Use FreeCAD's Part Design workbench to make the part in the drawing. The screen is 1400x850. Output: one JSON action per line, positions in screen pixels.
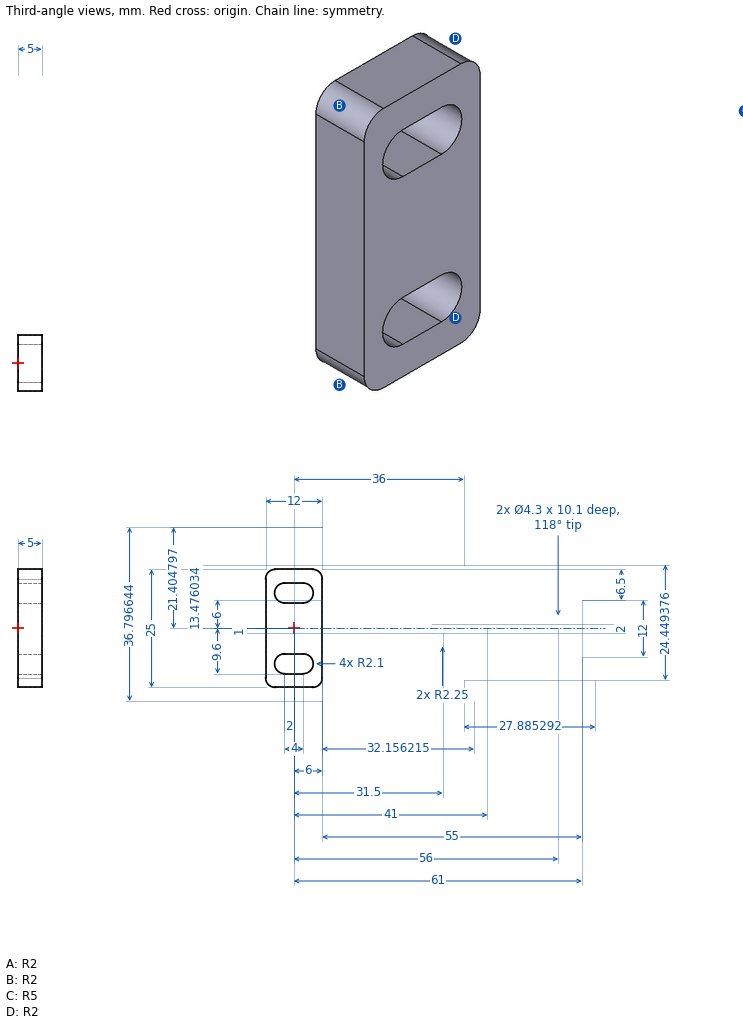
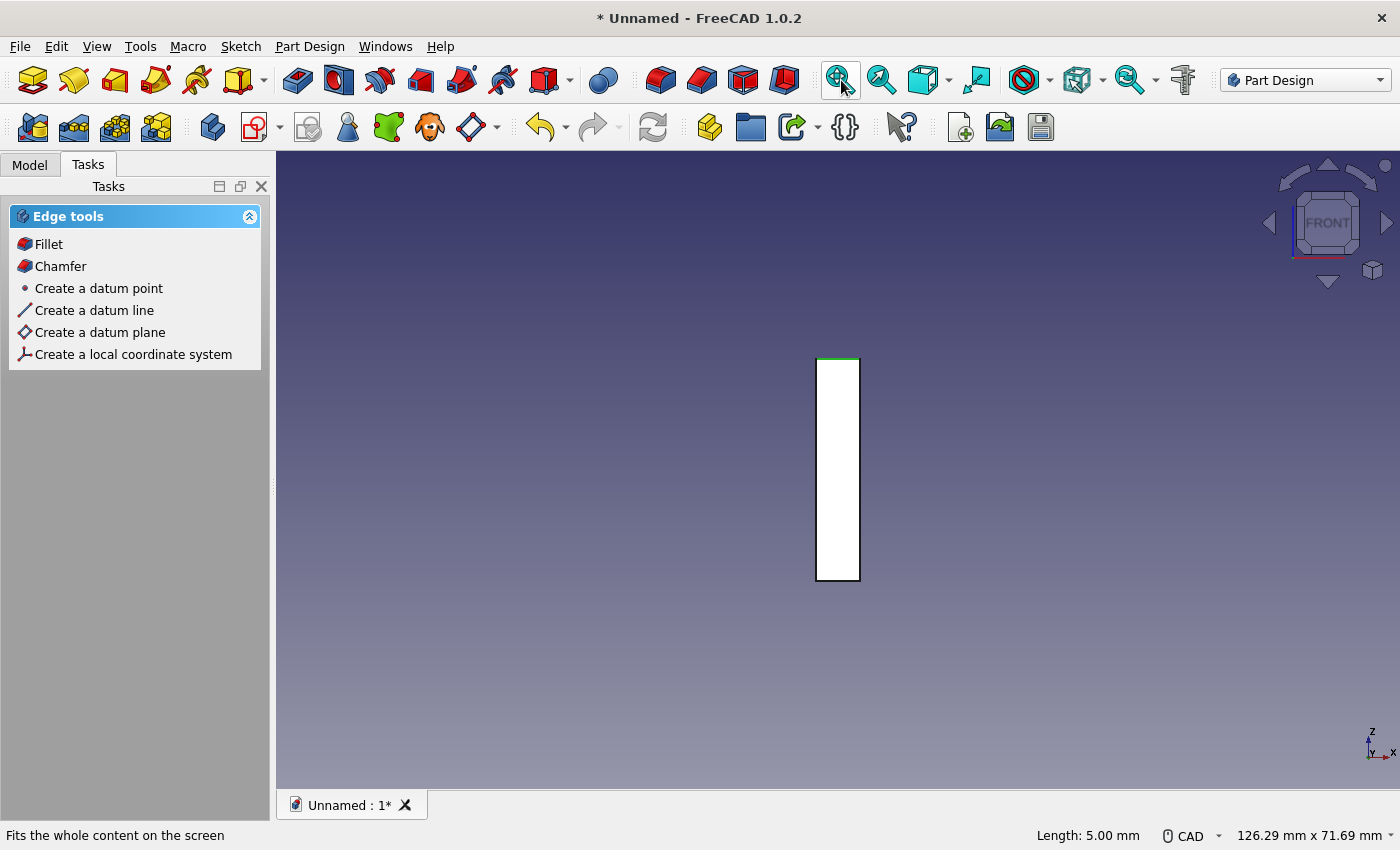
{"action": "left_click", "coordinate": [838, 580], "text": "ctrl"}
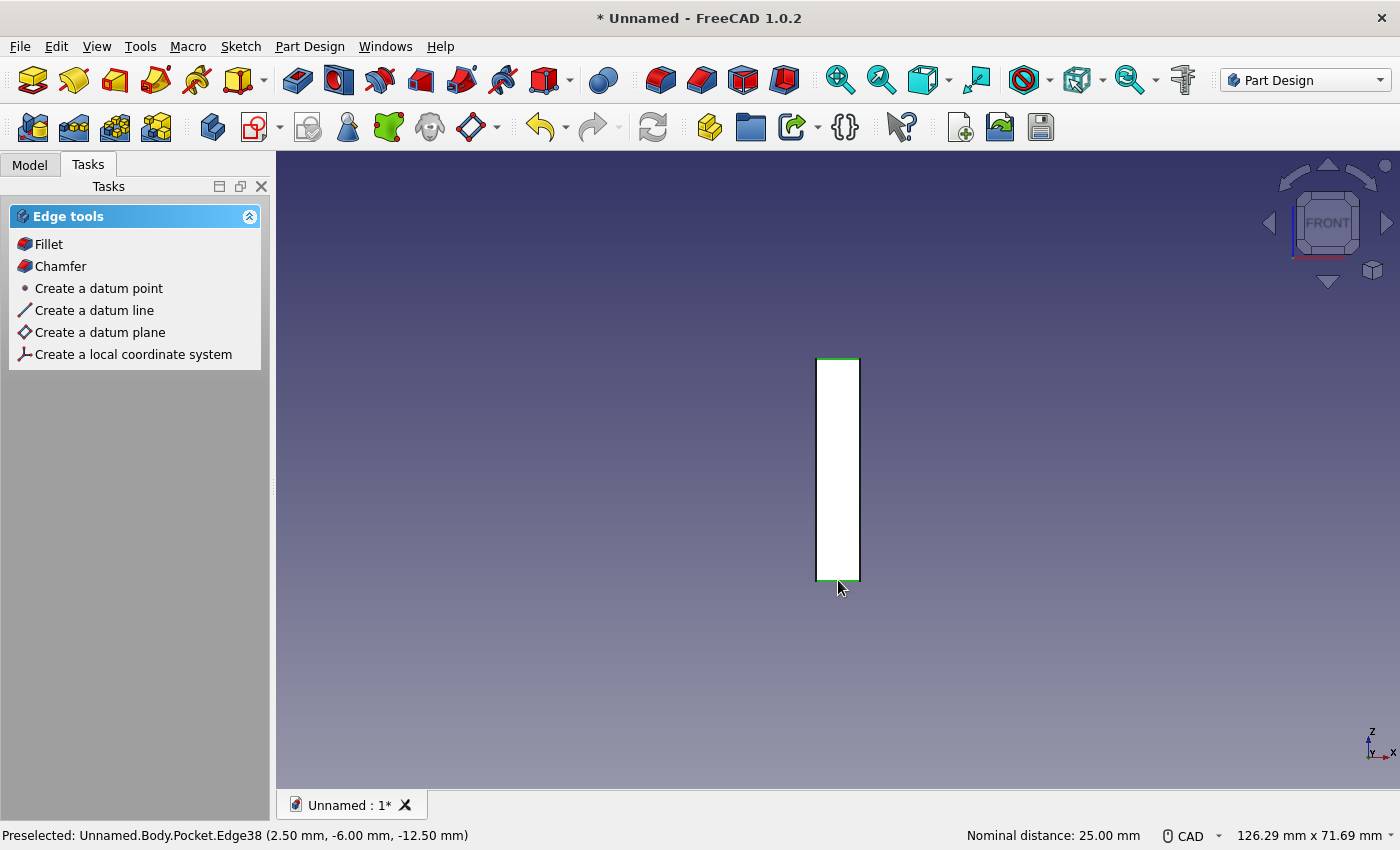
{"action": "left_click", "coordinate": [661, 80]}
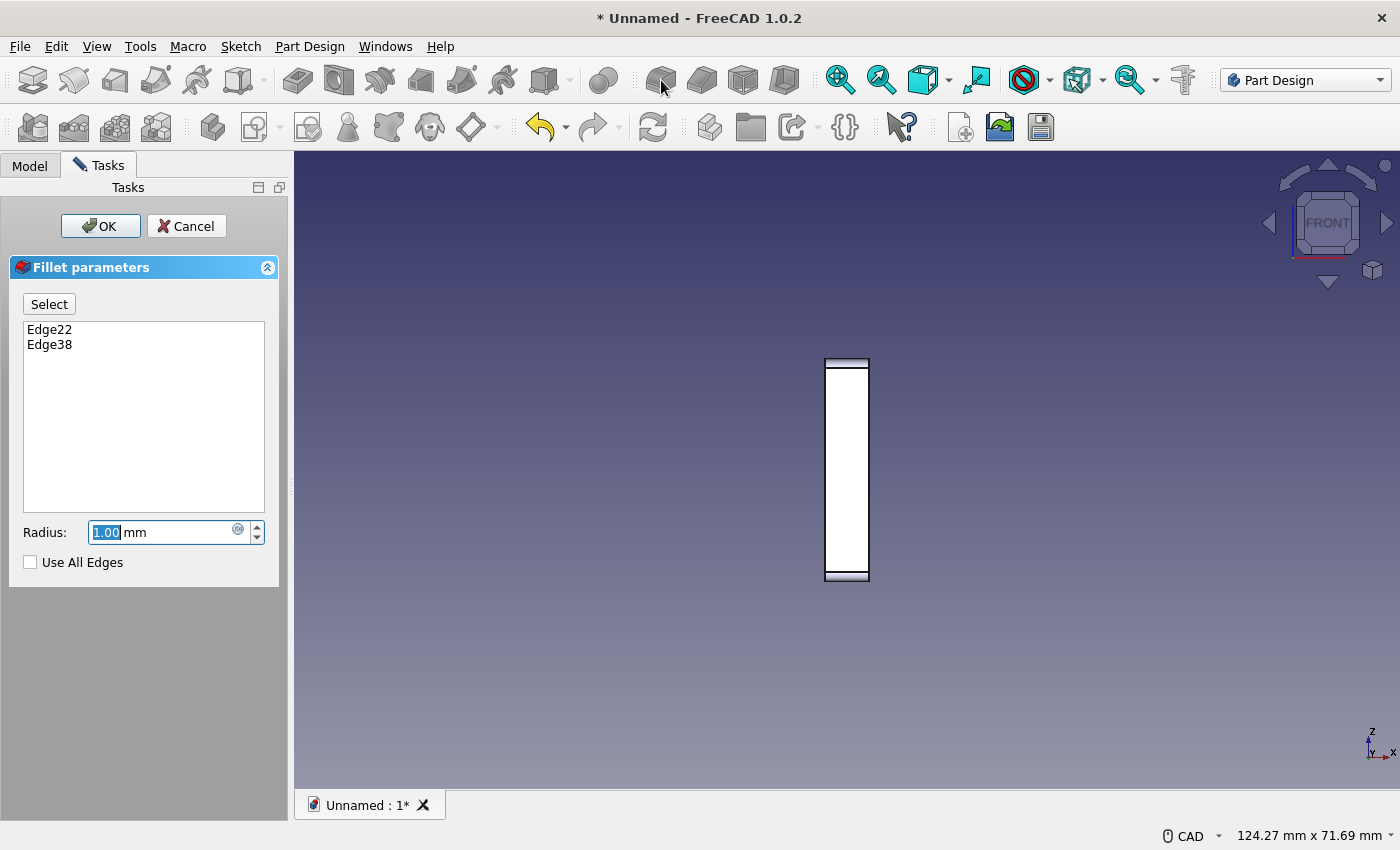
{"action": "type", "text": "2"}
{"action": "key", "text": "Tab"}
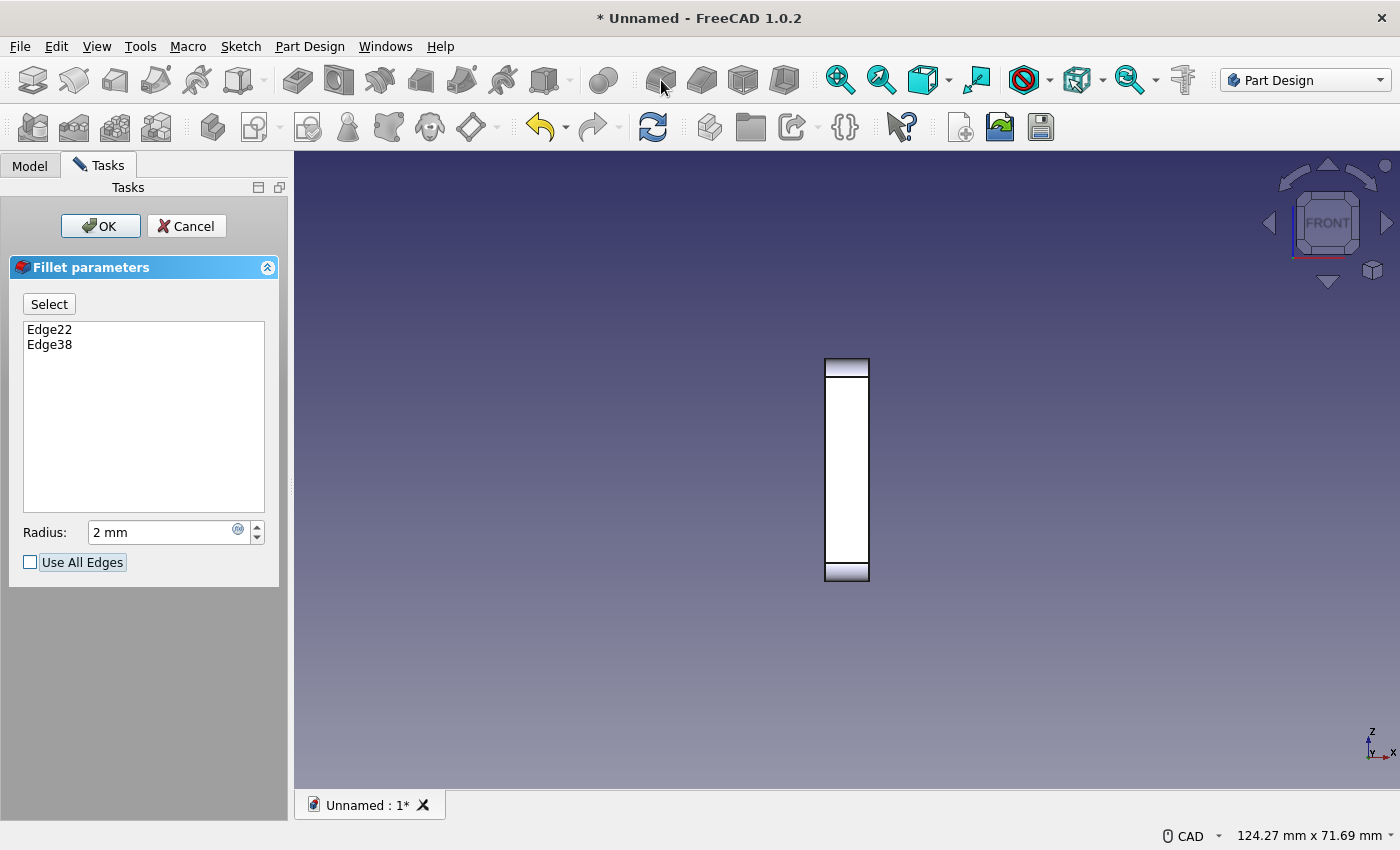
{"action": "left_click", "coordinate": [101, 226]}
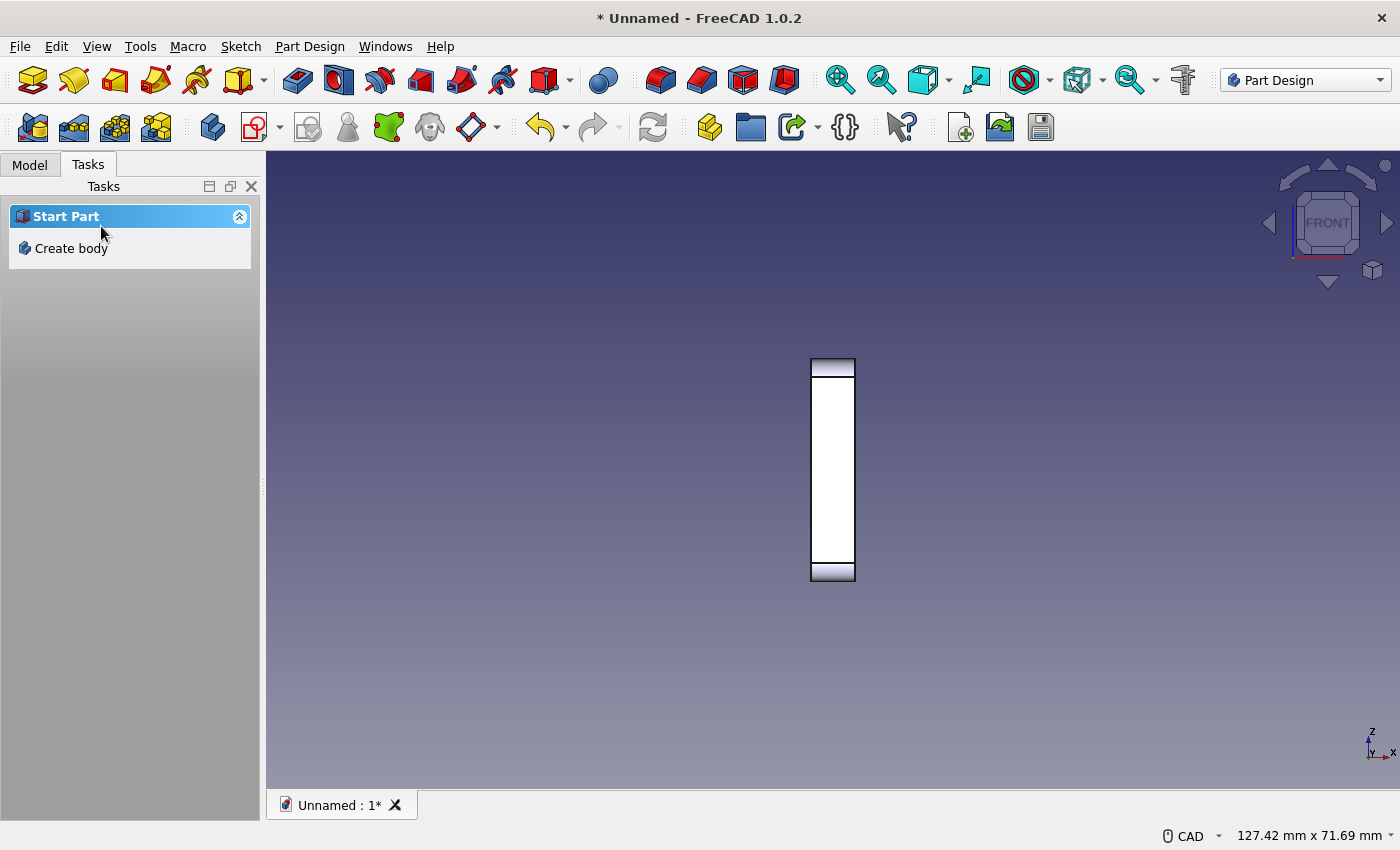
{"action": "left_click", "coordinate": [841, 80]}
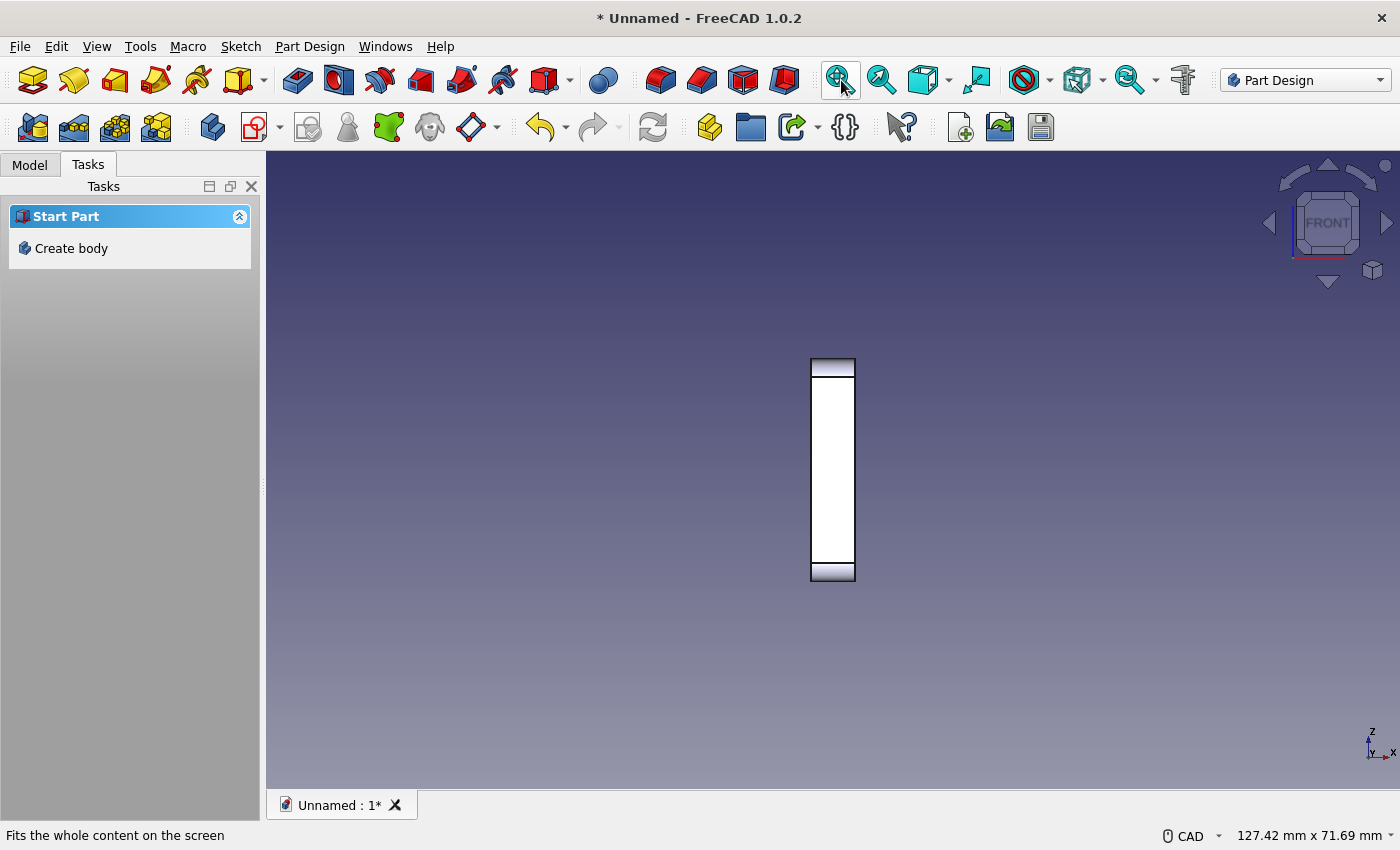
{"action": "left_click", "coordinate": [254, 128]}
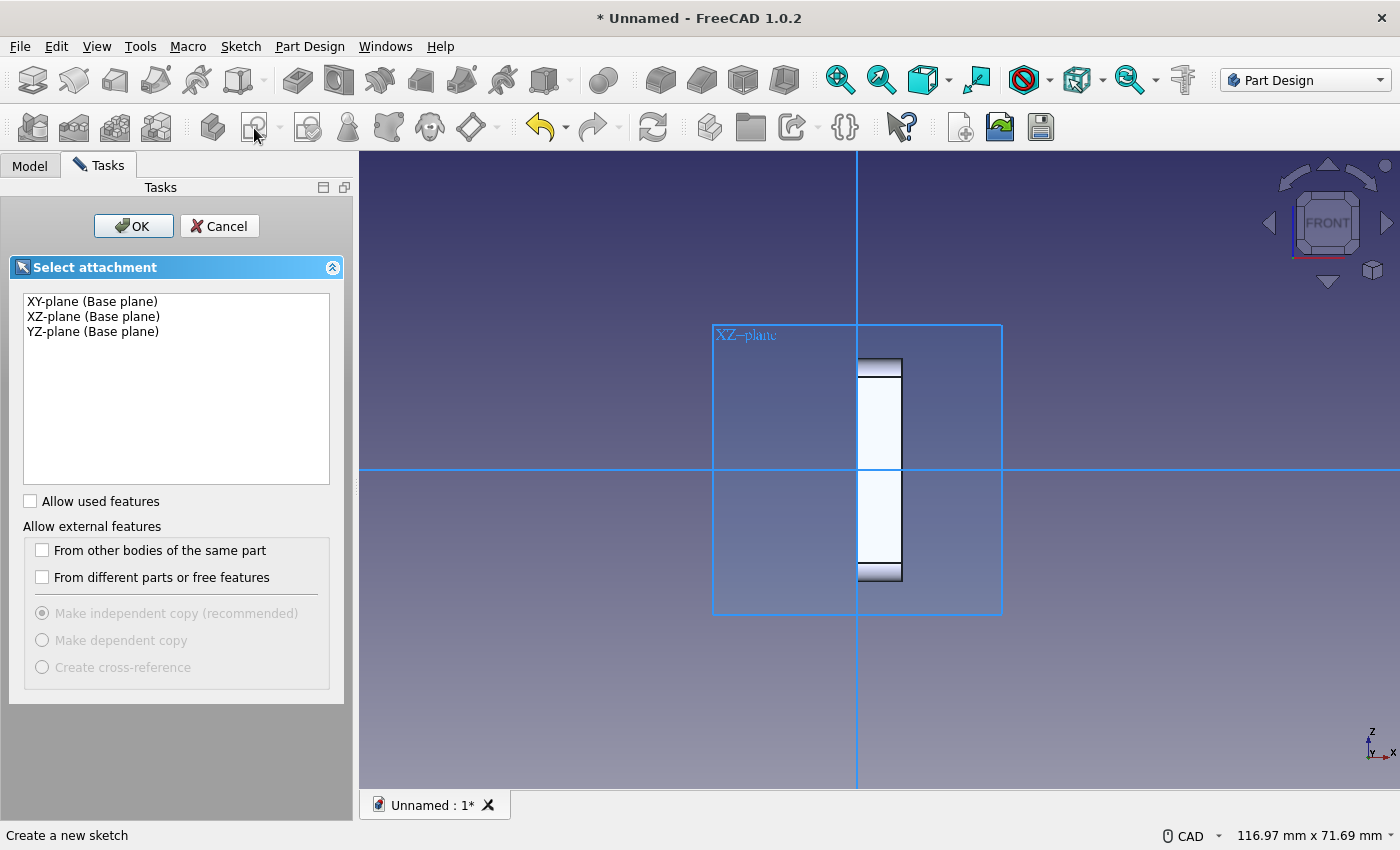
{"action": "left_click", "coordinate": [84, 332]}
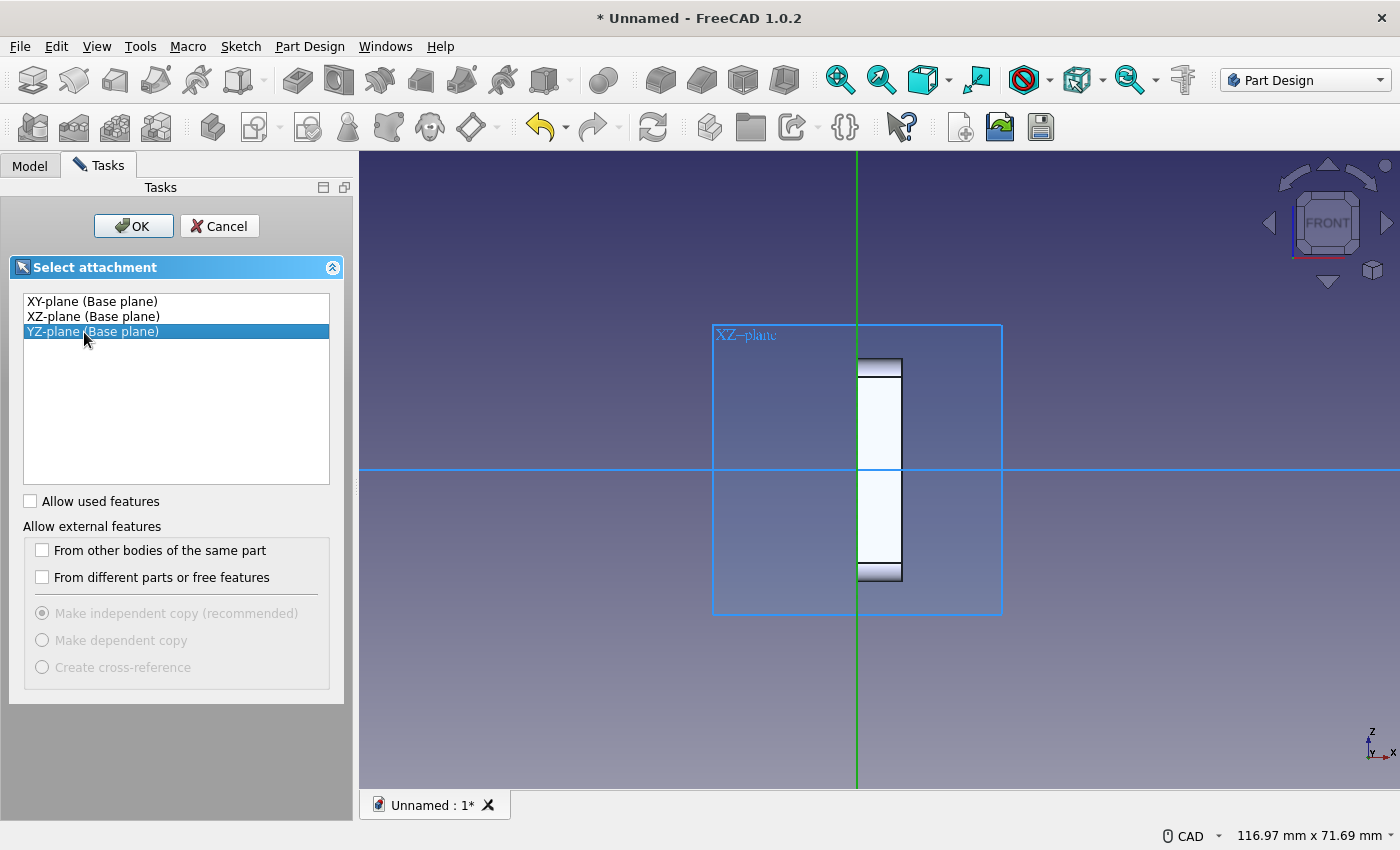
{"action": "left_click", "coordinate": [134, 226]}